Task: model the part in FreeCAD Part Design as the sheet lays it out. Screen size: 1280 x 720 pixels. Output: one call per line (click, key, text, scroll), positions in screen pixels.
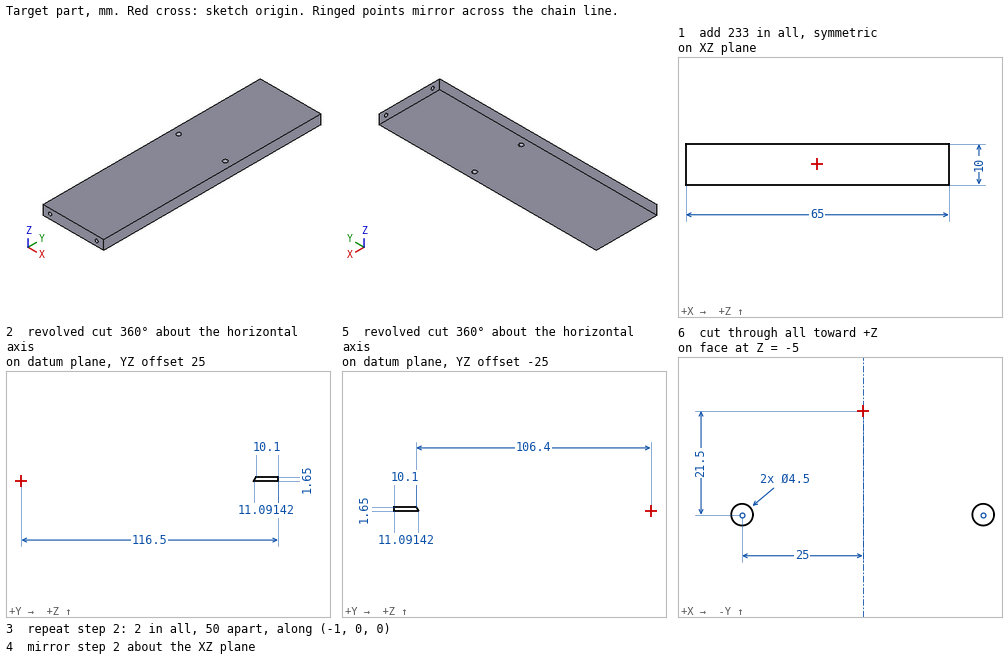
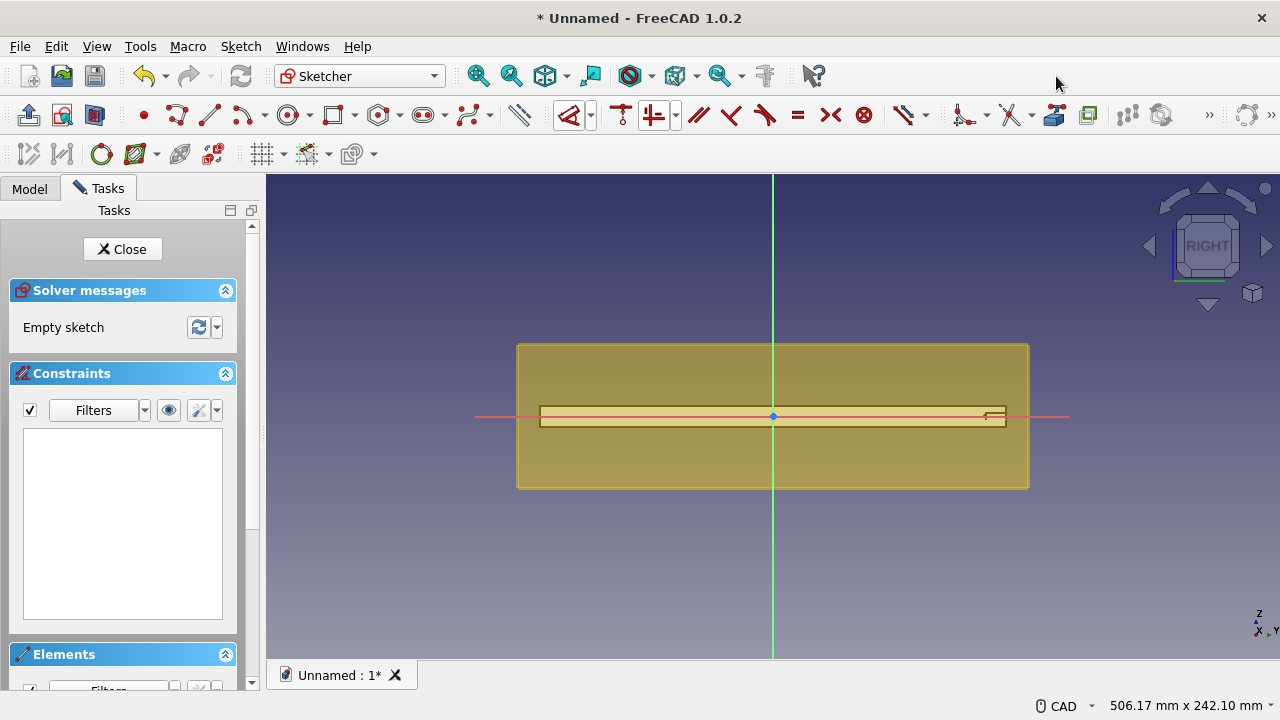
scroll(543, 415, up, 15)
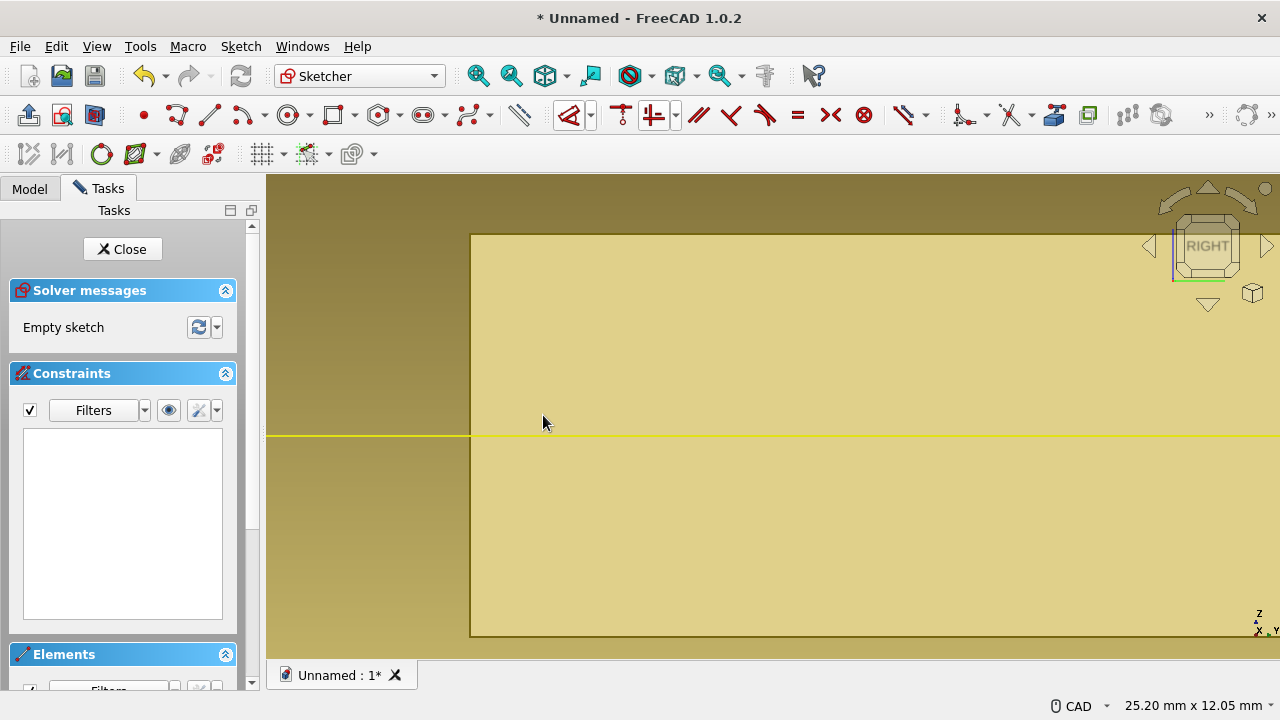
key(g)
key(m)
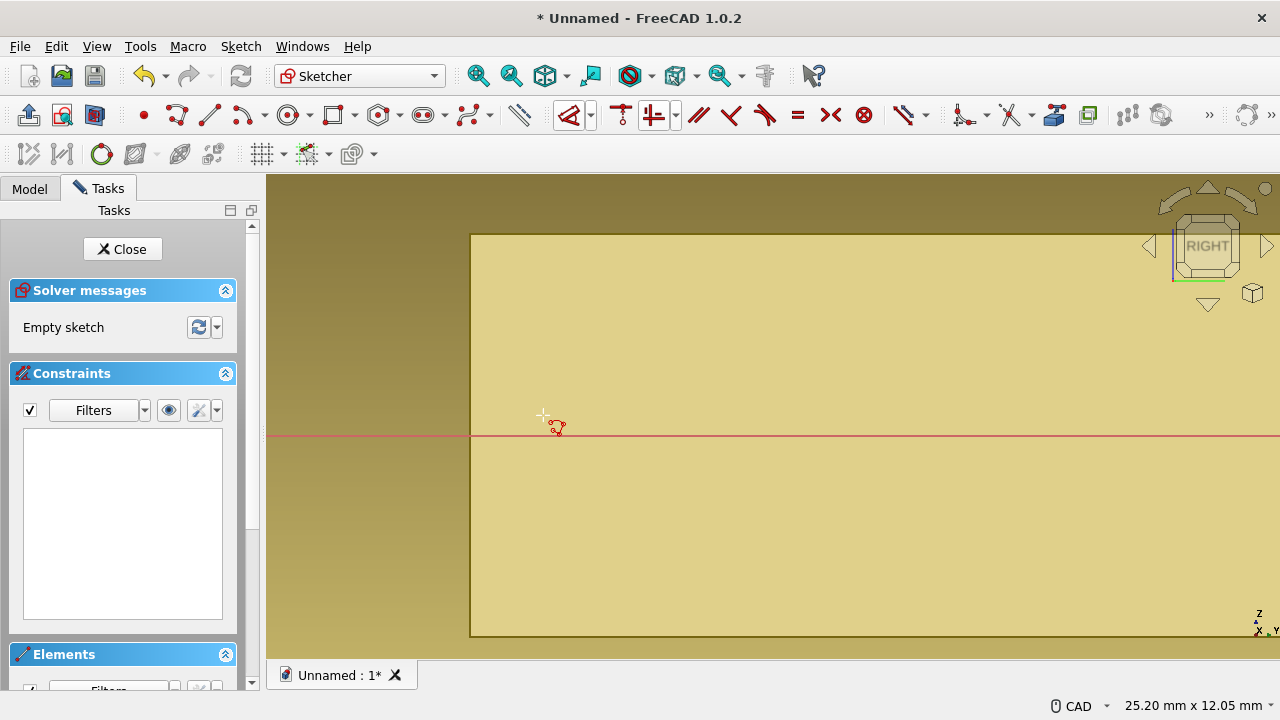
click(916, 436)
click(876, 369)
click(470, 369)
click(470, 427)
click(916, 436)
key(Escape)
key(Escape)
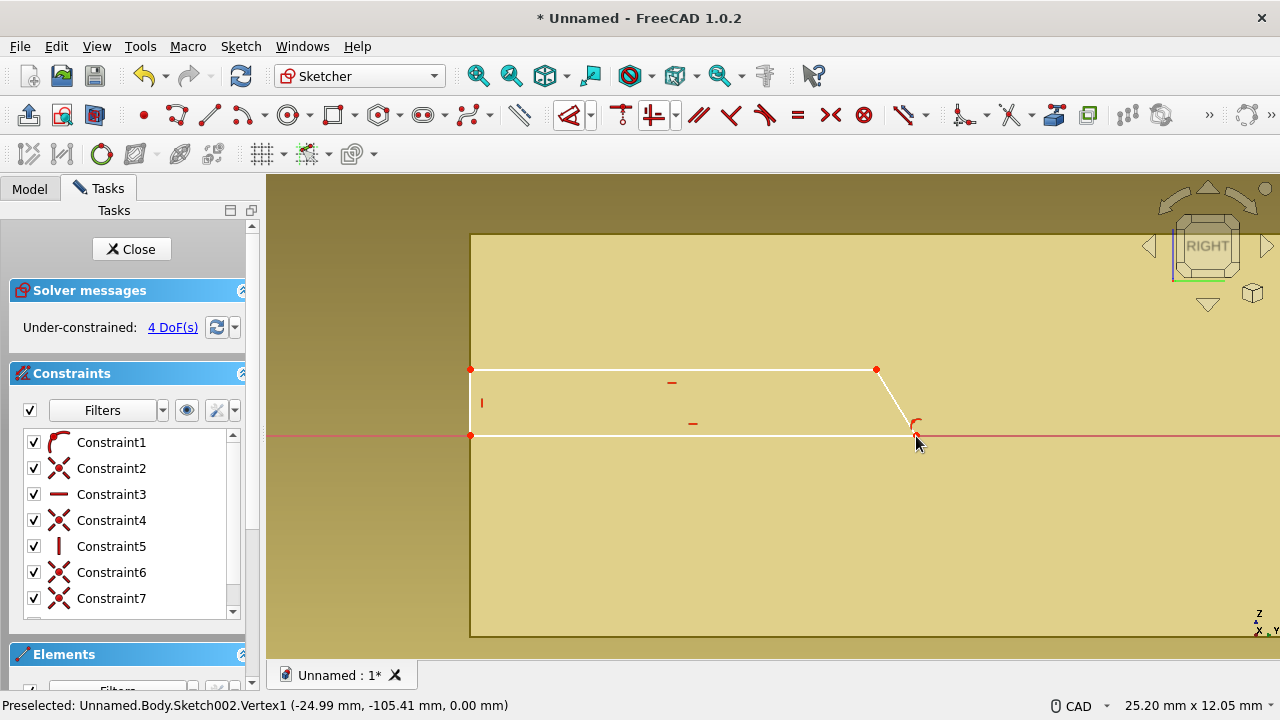
key(d)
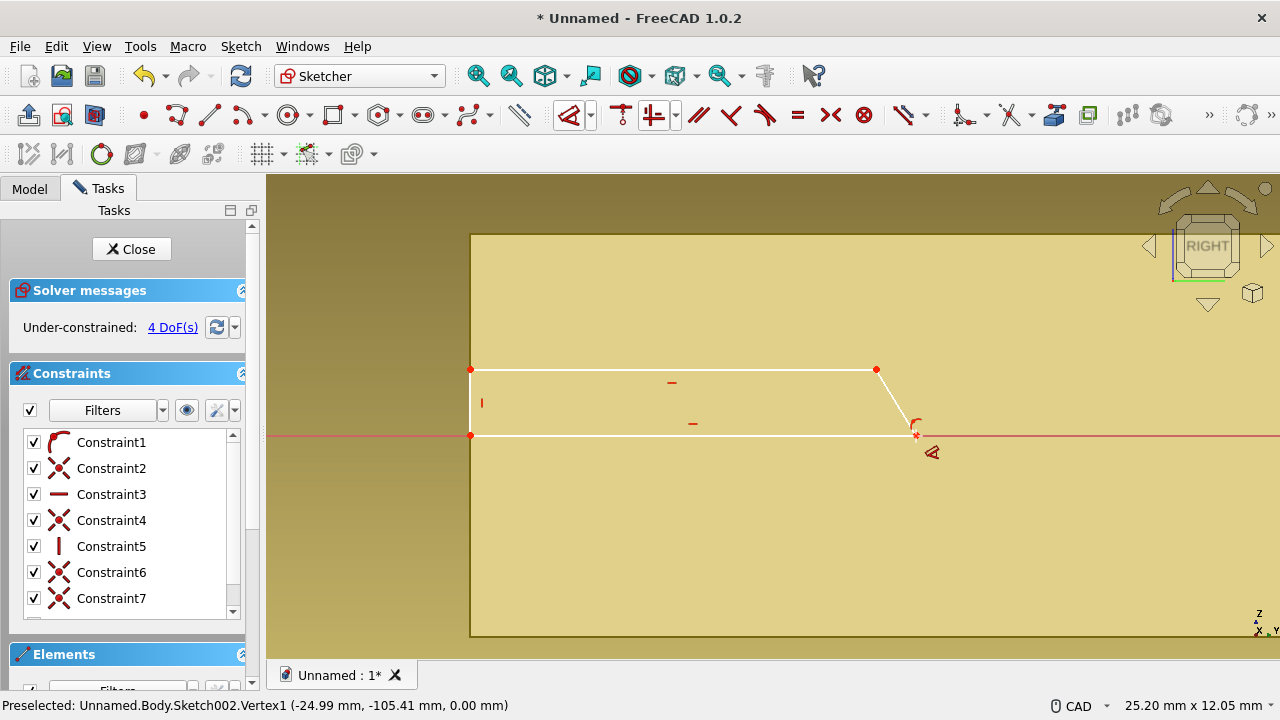
click(754, 370)
click(673, 336)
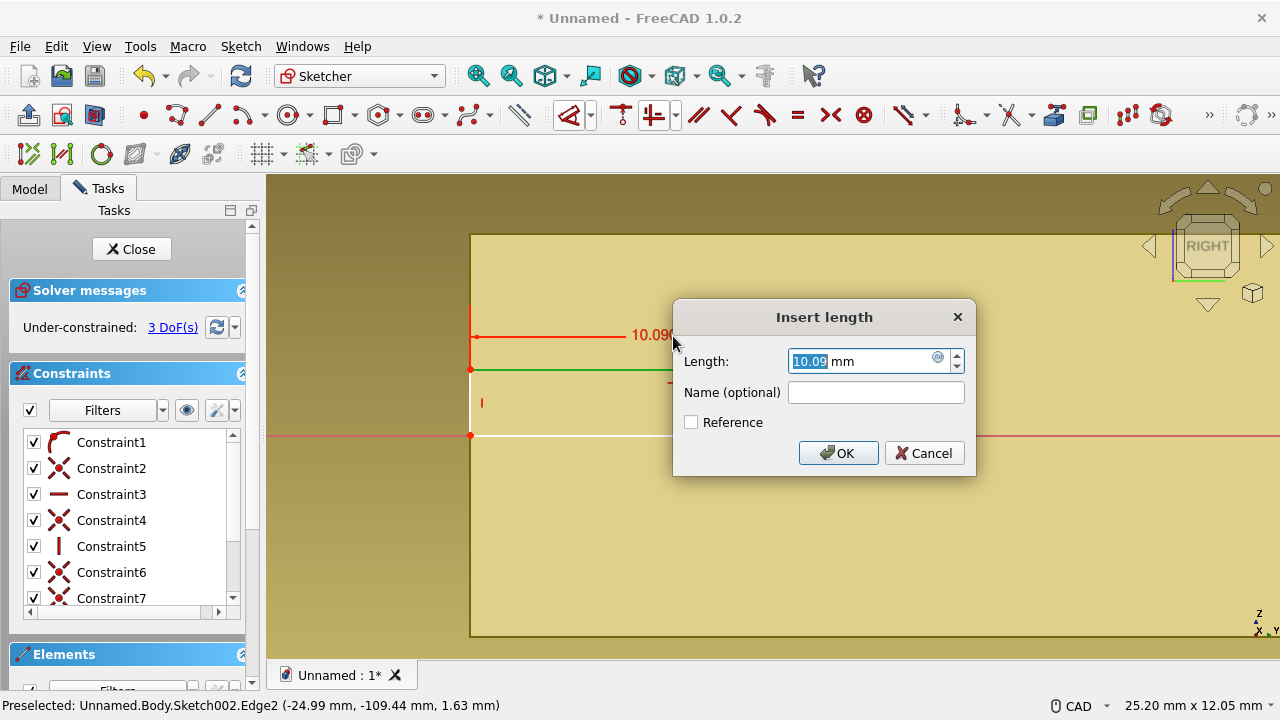
text(10.1)
key(Return)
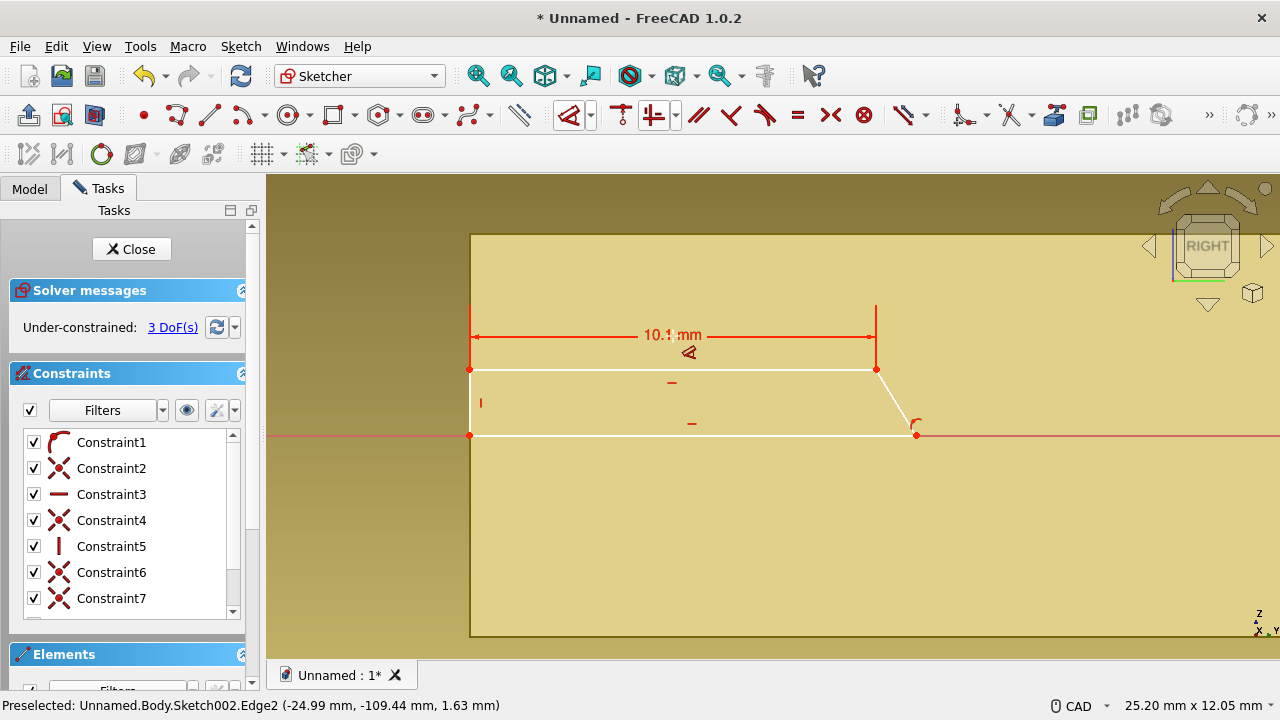
click(470, 390)
click(436, 403)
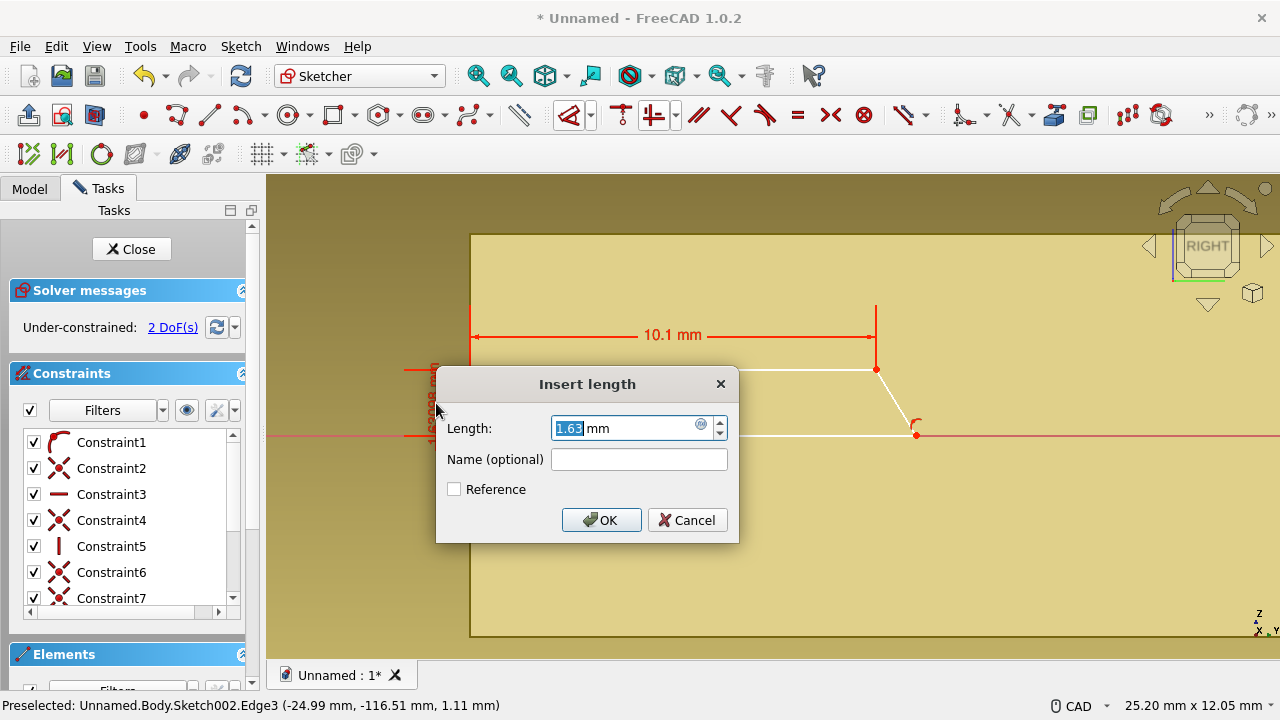
text(1.65)
key(Return)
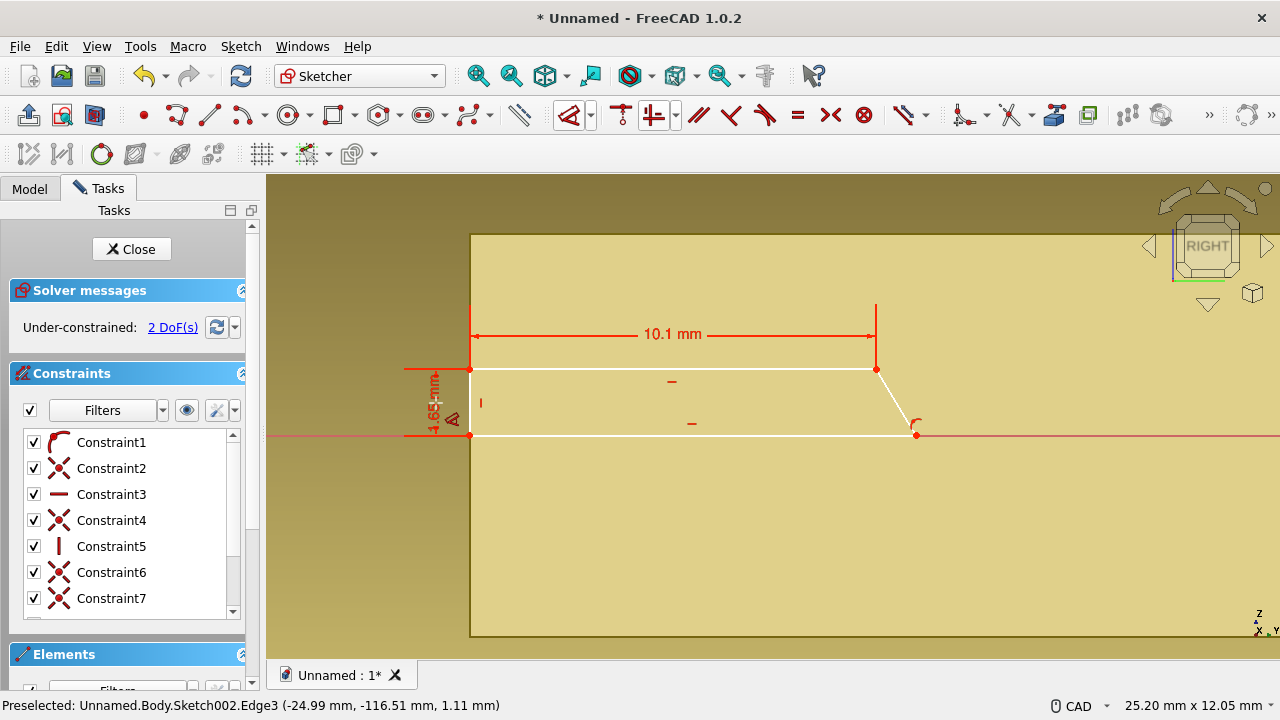
click(876, 369)
click(995, 335)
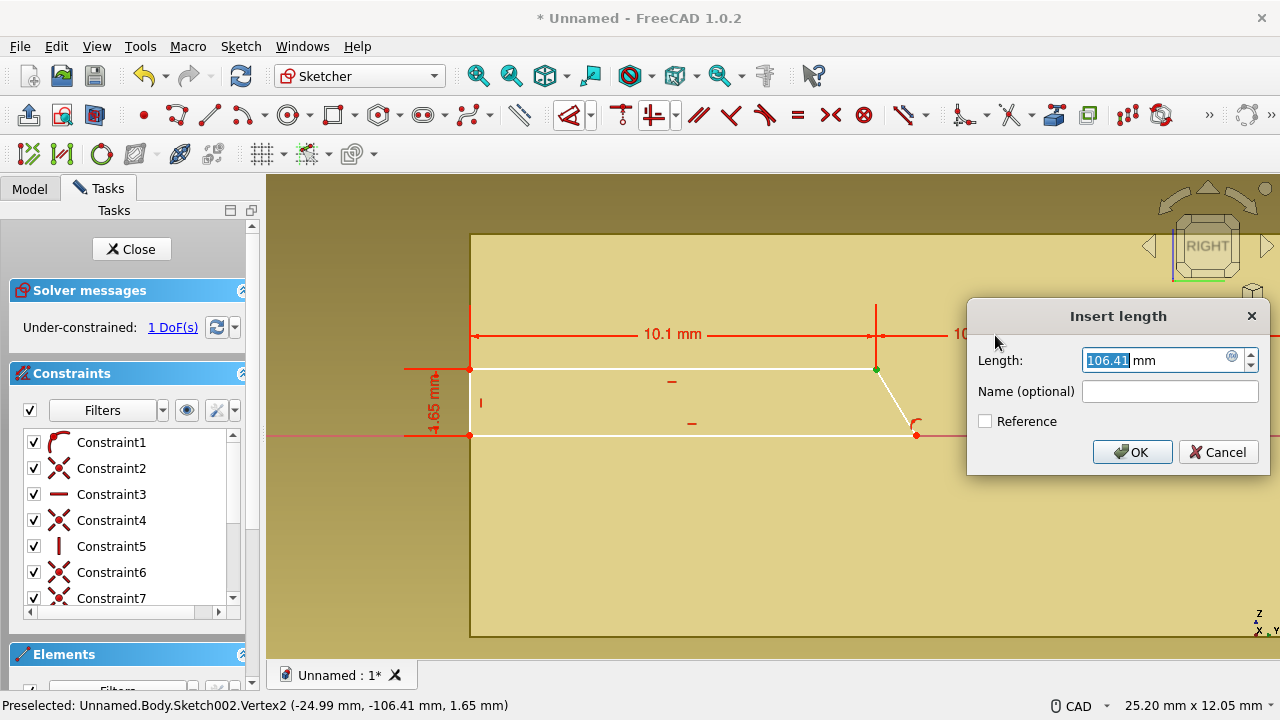
text(106.4)
key(Return)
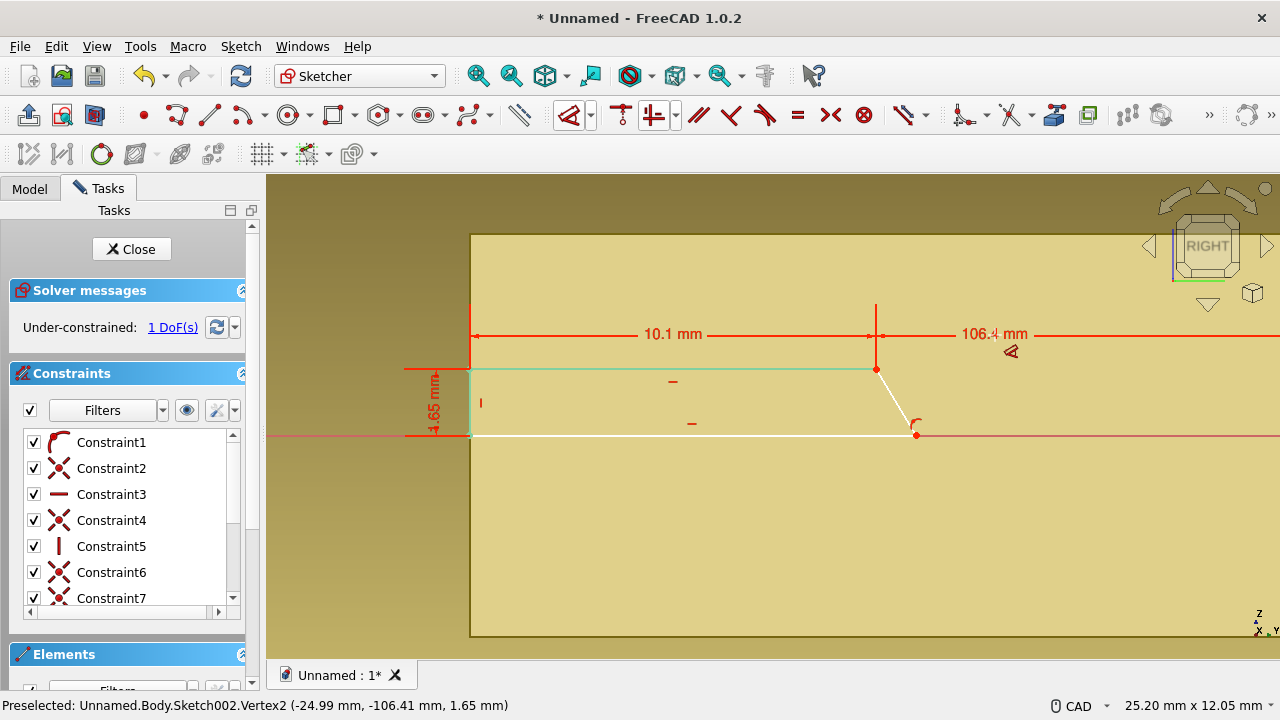
click(604, 436)
click(693, 470)